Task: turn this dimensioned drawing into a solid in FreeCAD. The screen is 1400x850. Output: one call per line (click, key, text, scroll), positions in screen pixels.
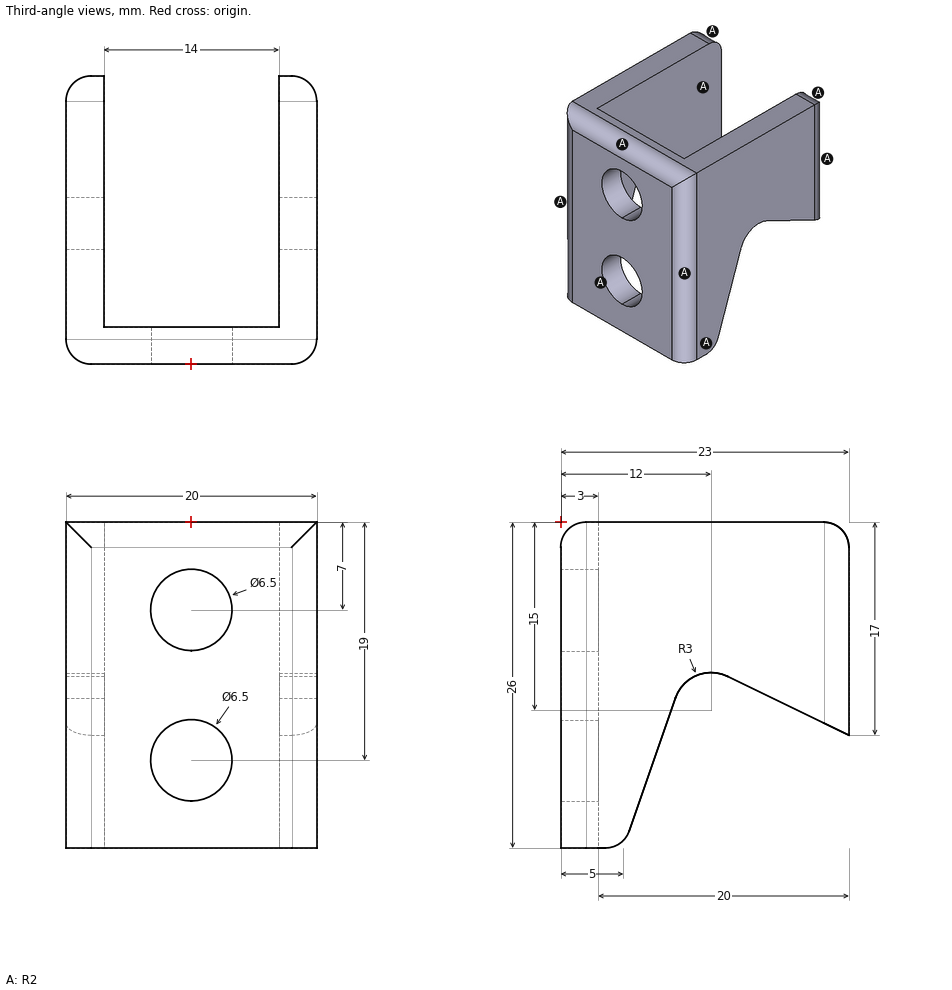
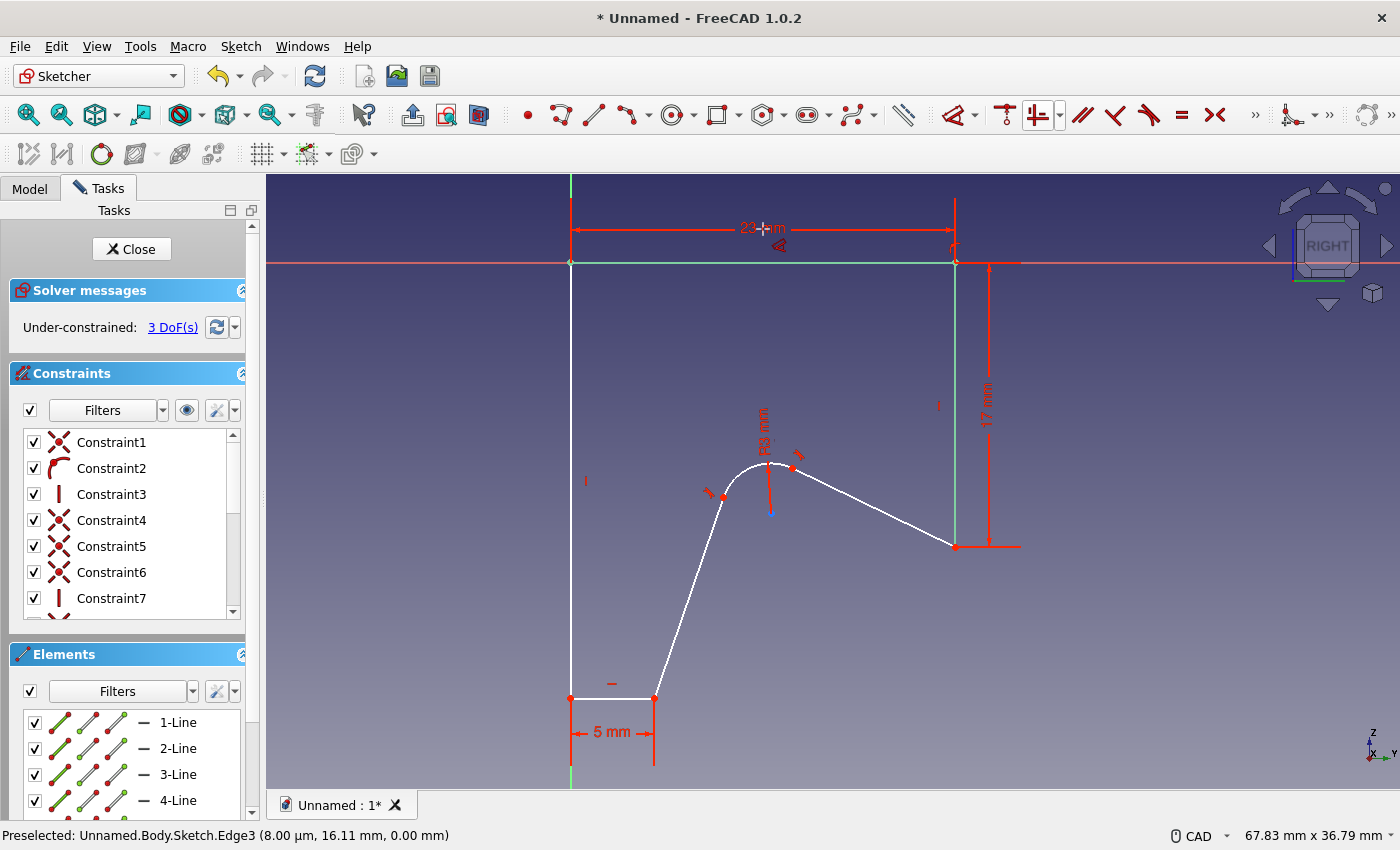
click(571, 394)
click(537, 481)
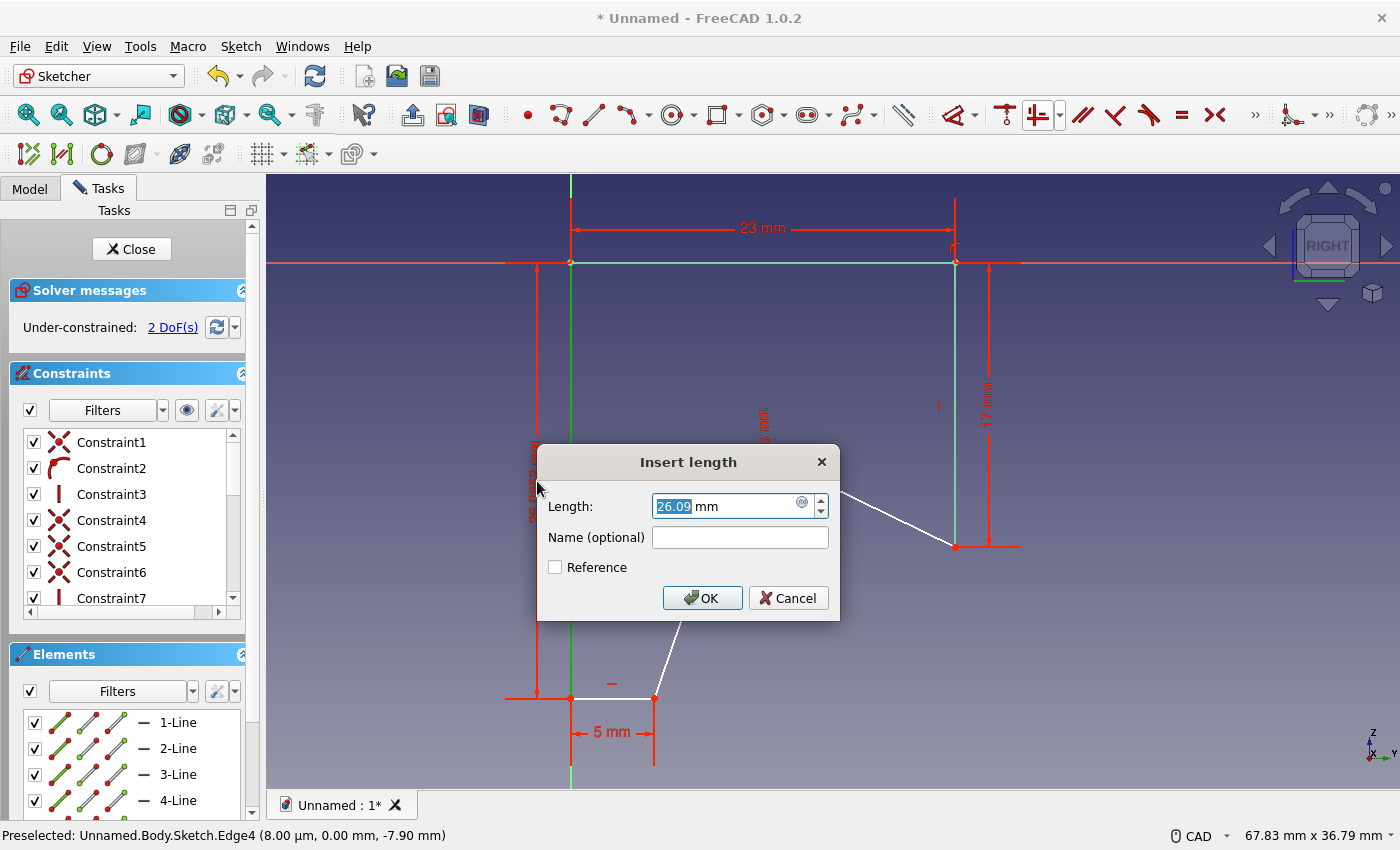
text(26)
key(Return)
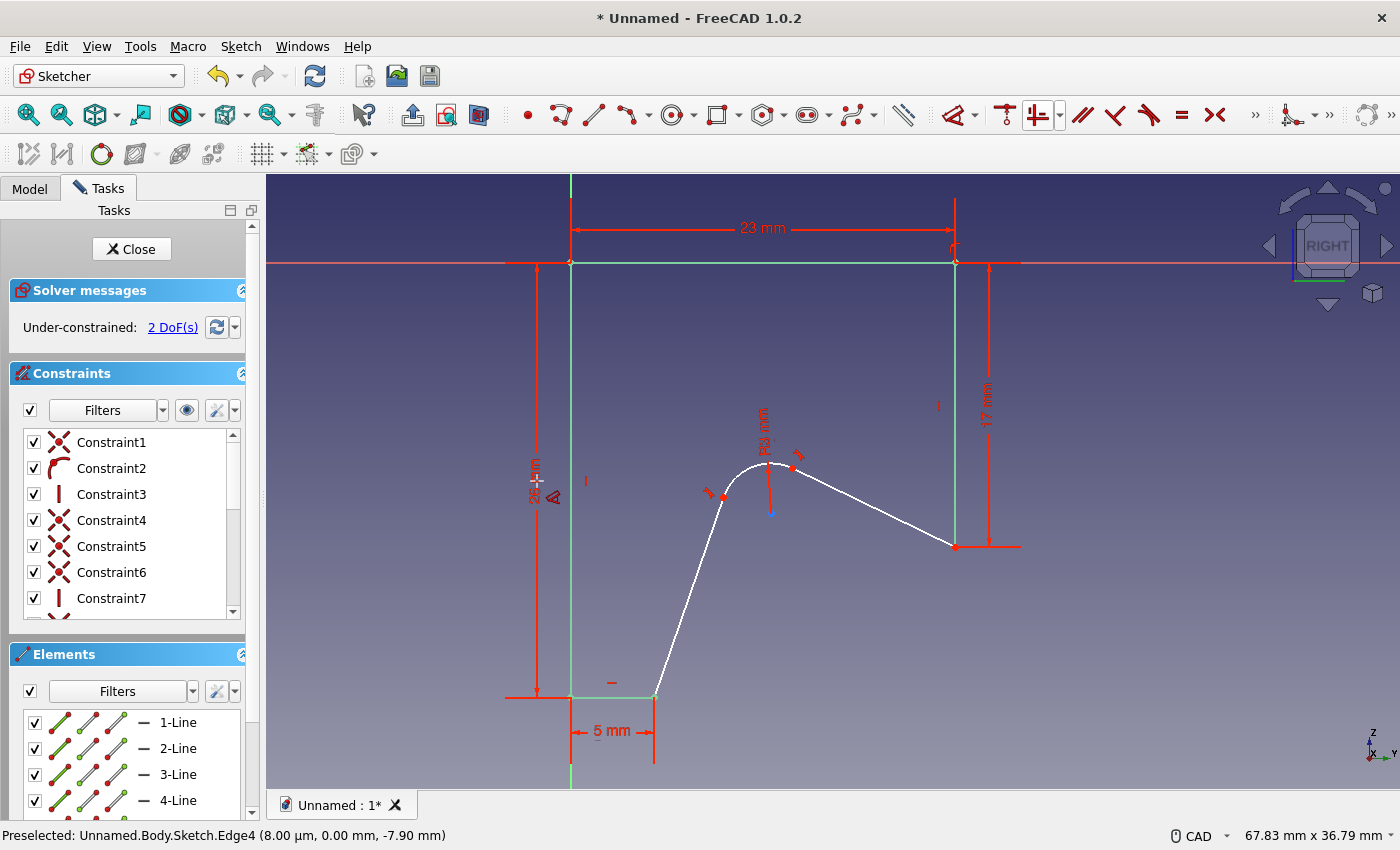
click(771, 514)
click(671, 229)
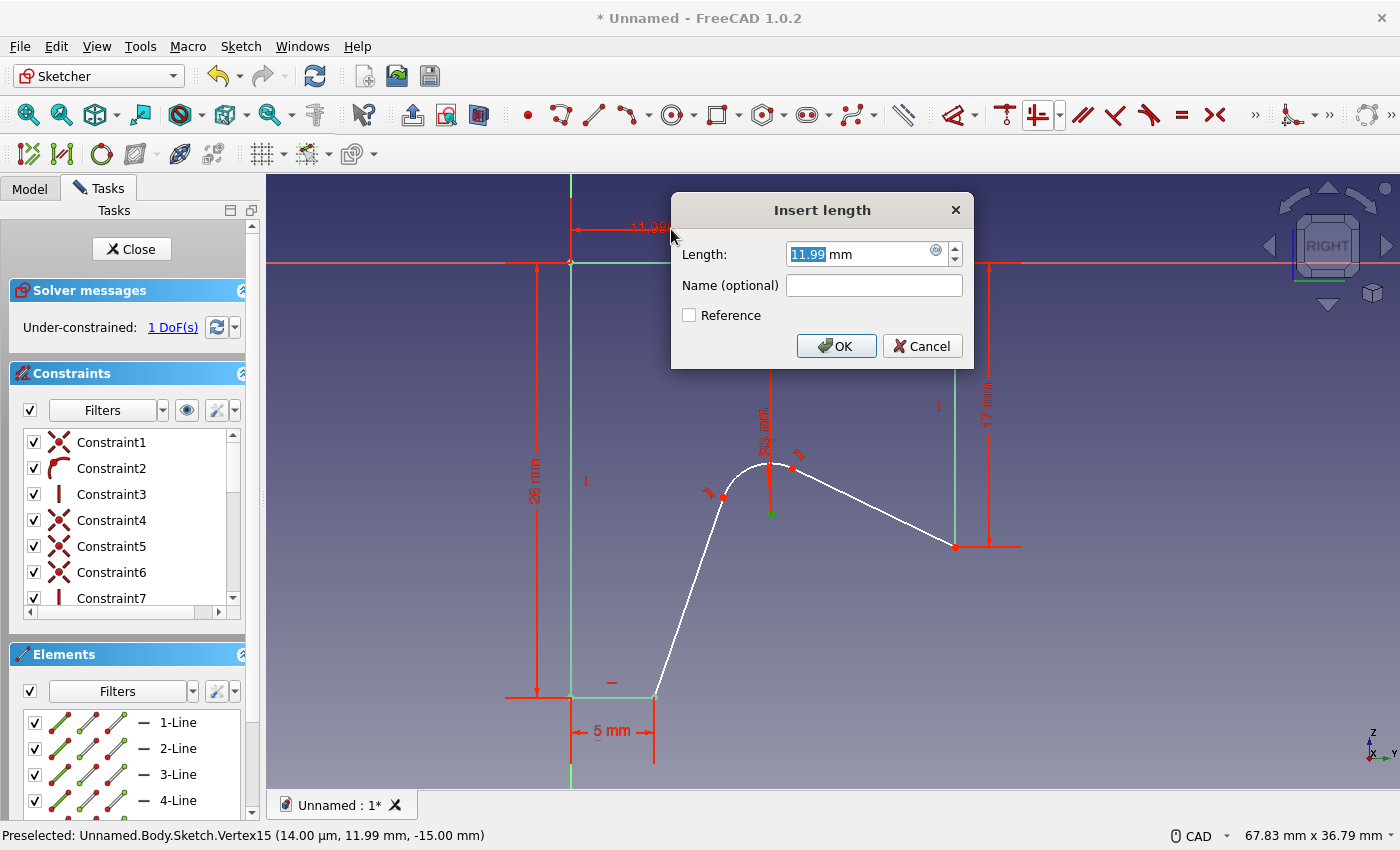
text(12)
key(Return)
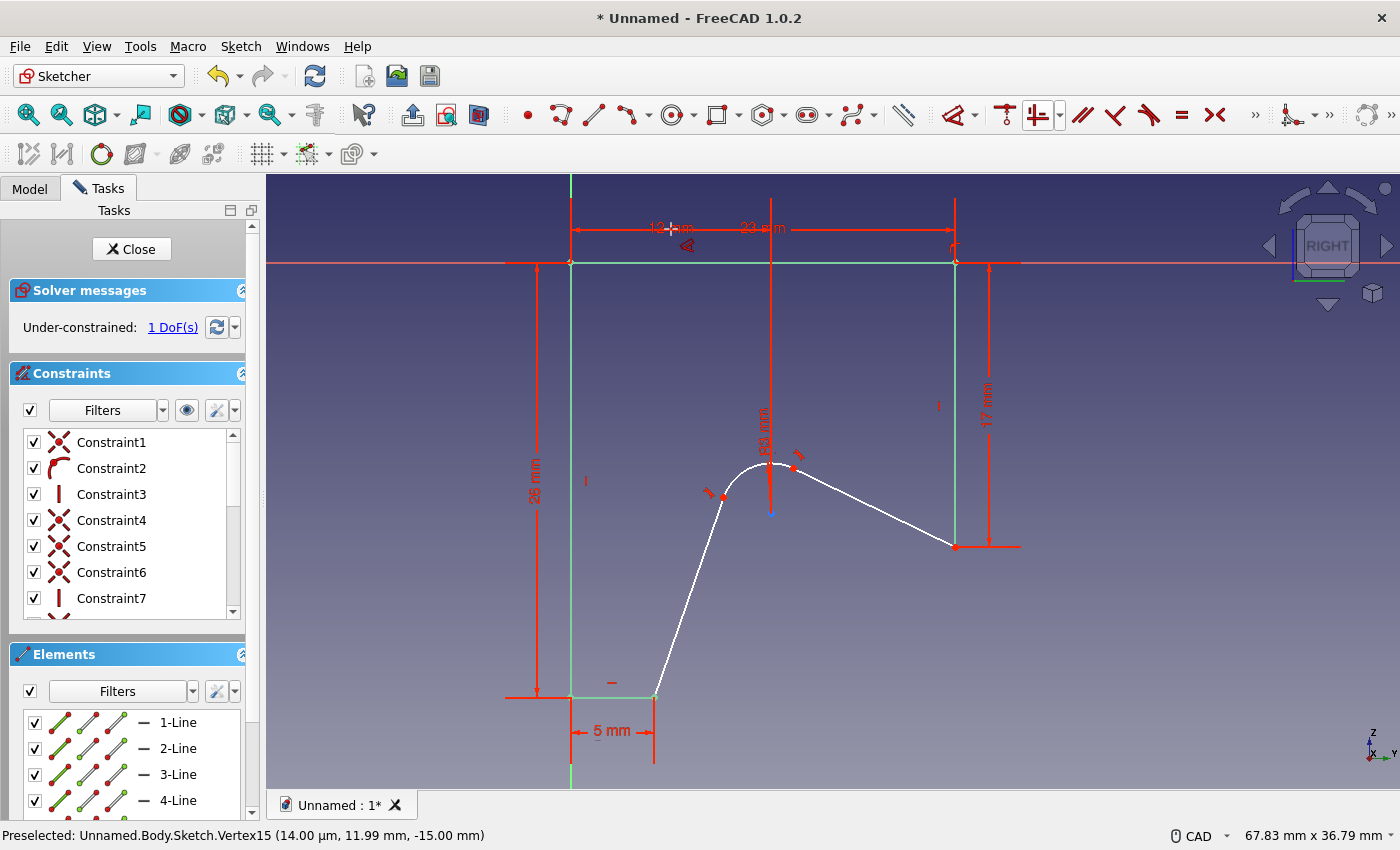
click(771, 514)
click(537, 388)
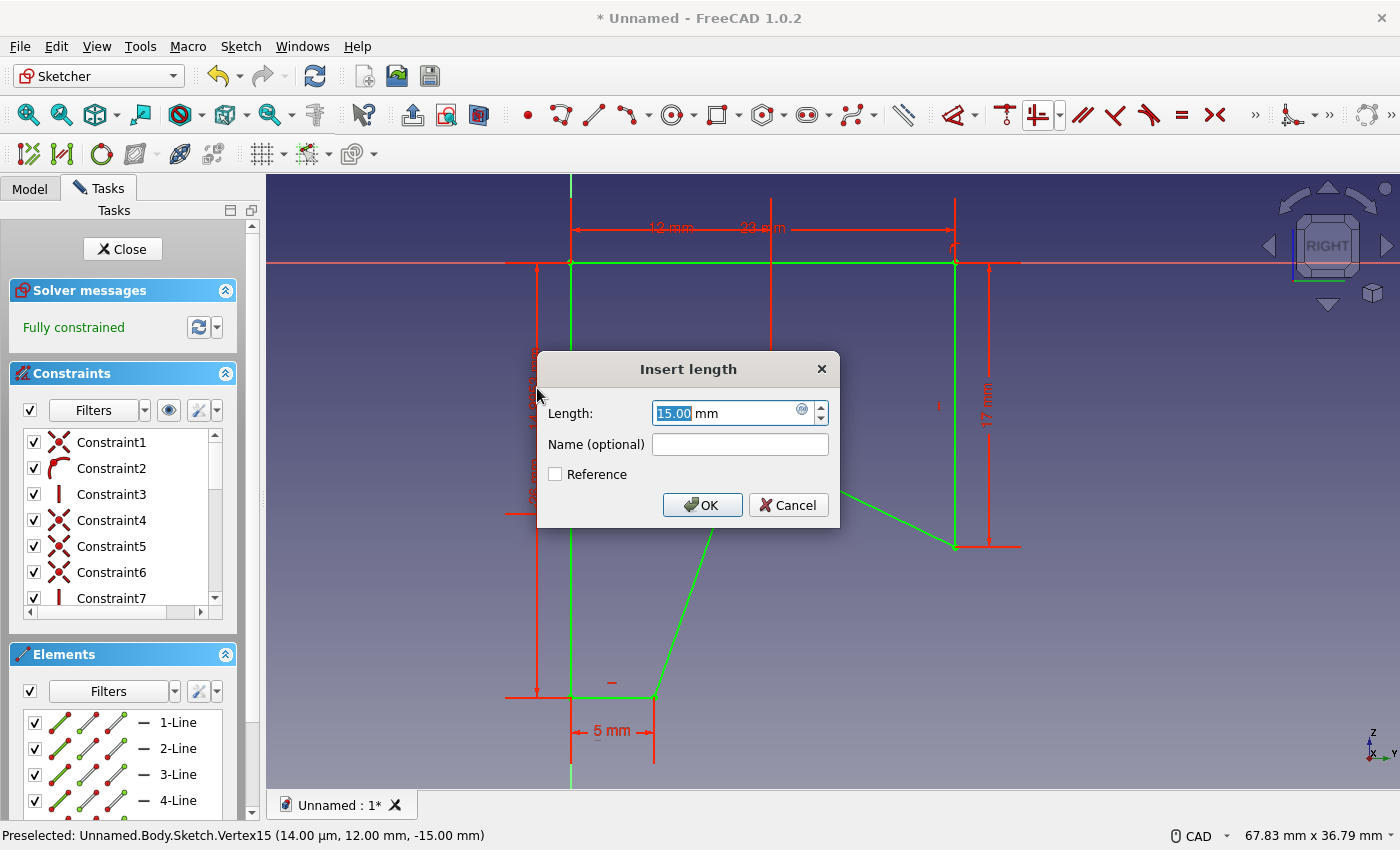
text(15)
key(Return)
key(Escape)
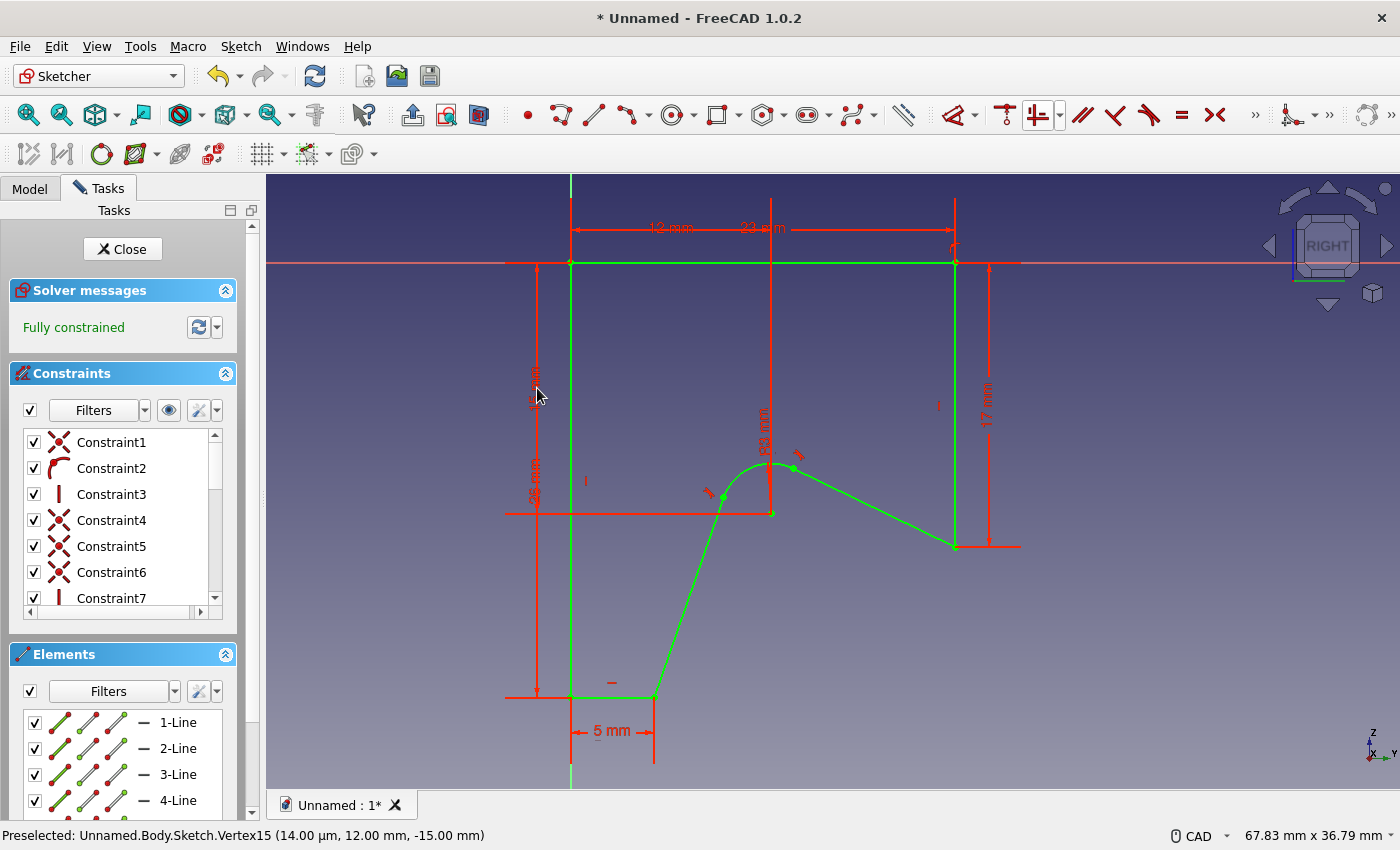
click(123, 249)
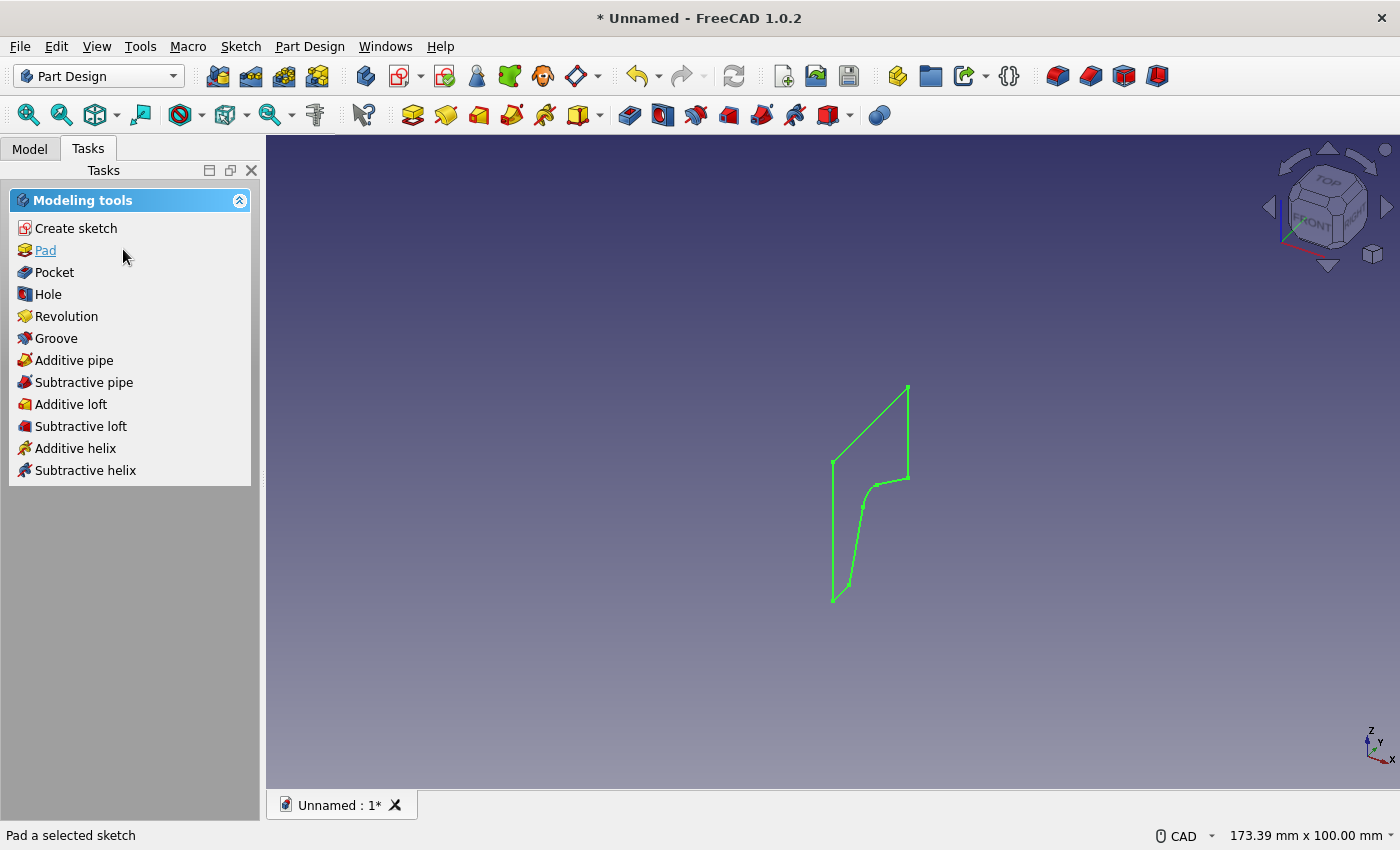
click(413, 116)